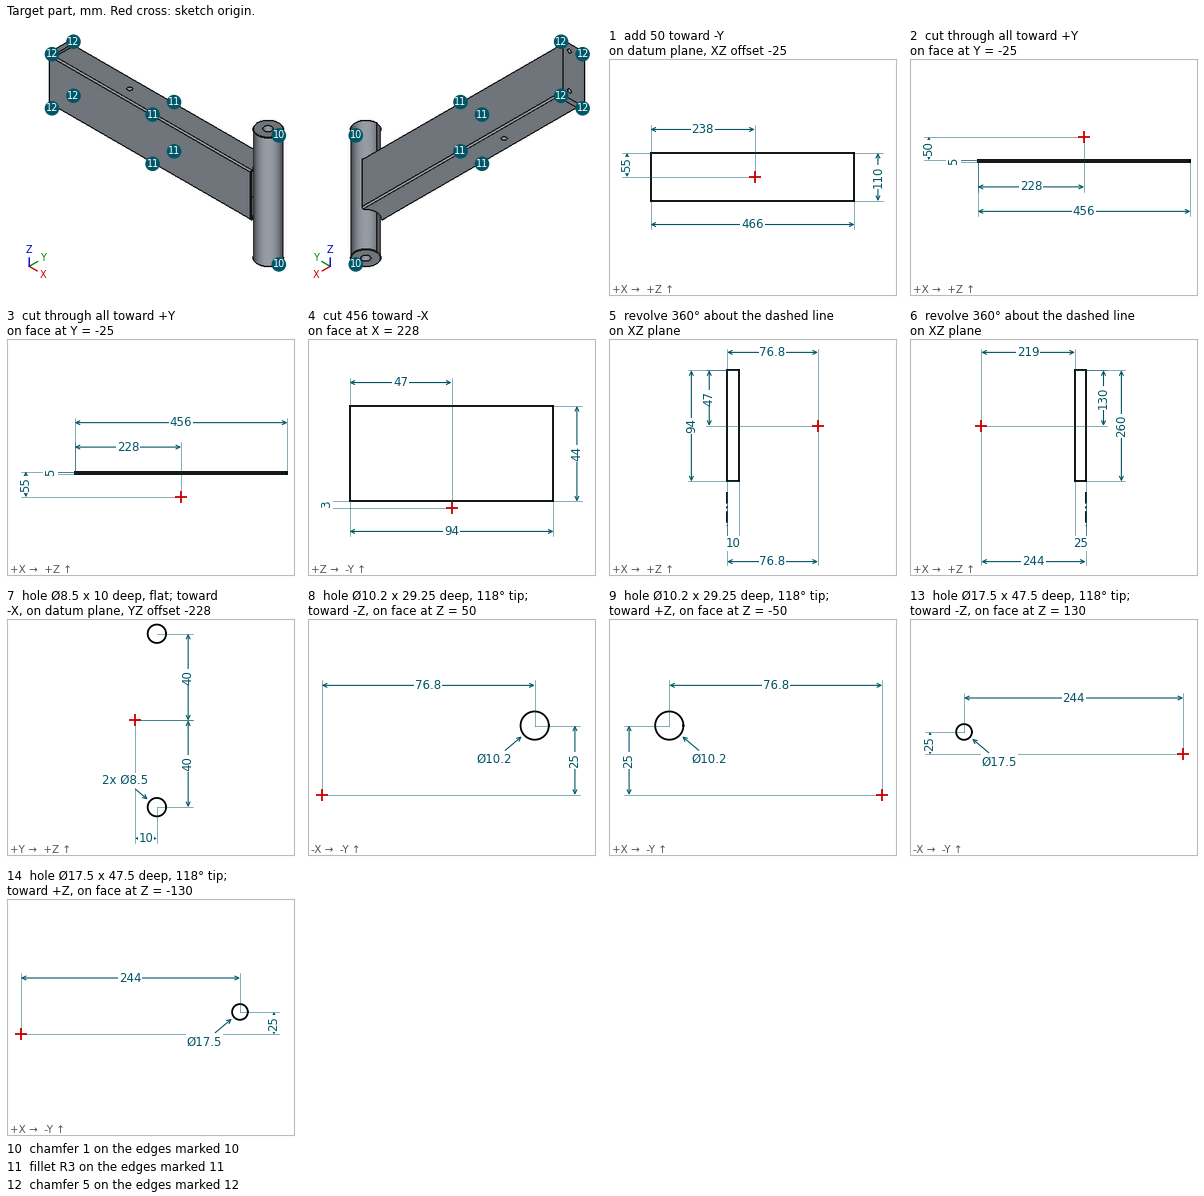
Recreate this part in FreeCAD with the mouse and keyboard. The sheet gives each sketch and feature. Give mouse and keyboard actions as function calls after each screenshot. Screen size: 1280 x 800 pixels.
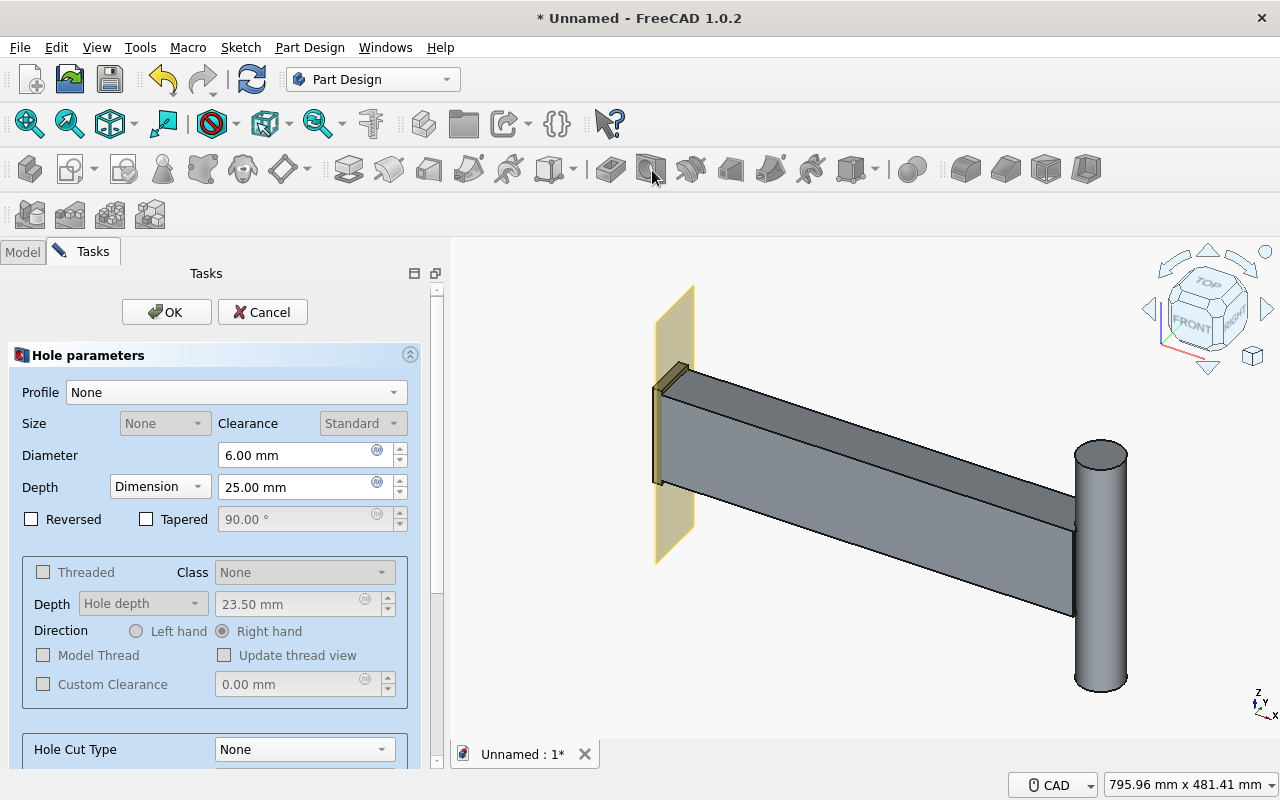
triple_click(305, 455)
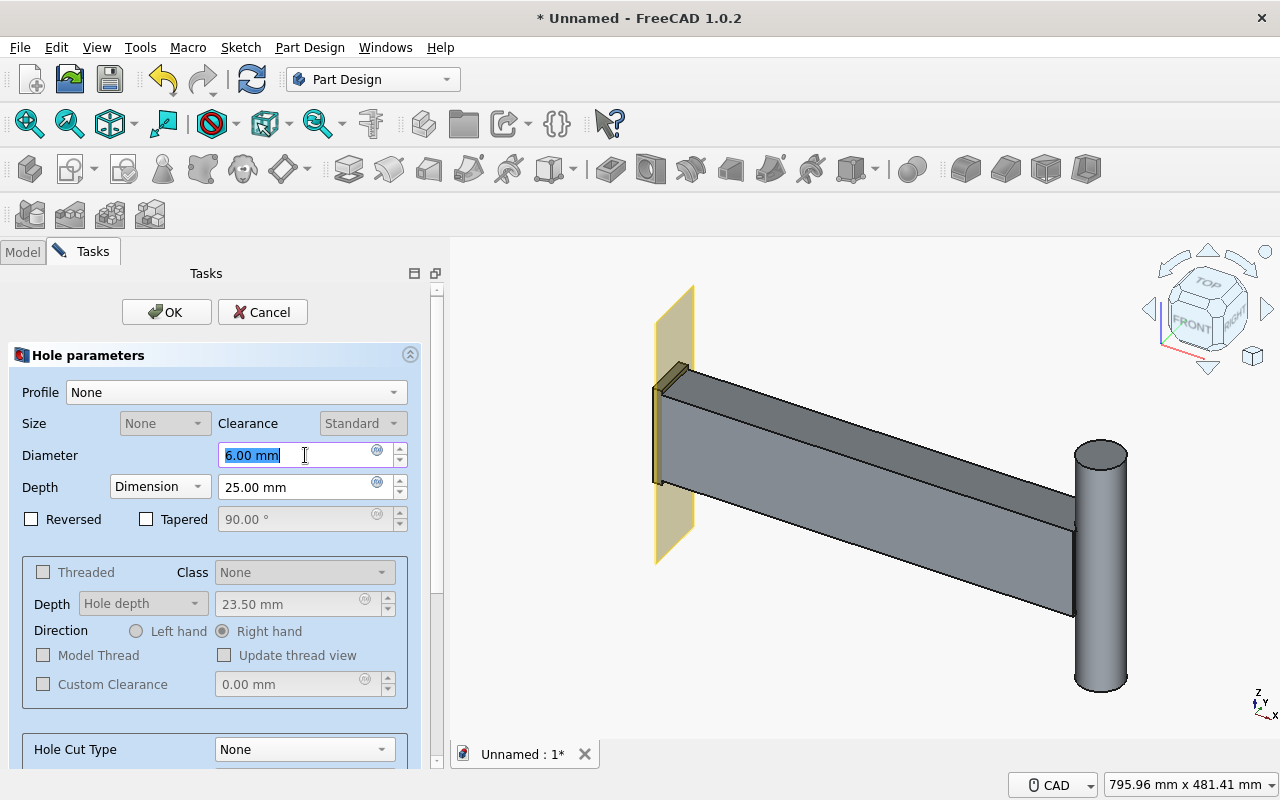
text(8.5)
key(Tab)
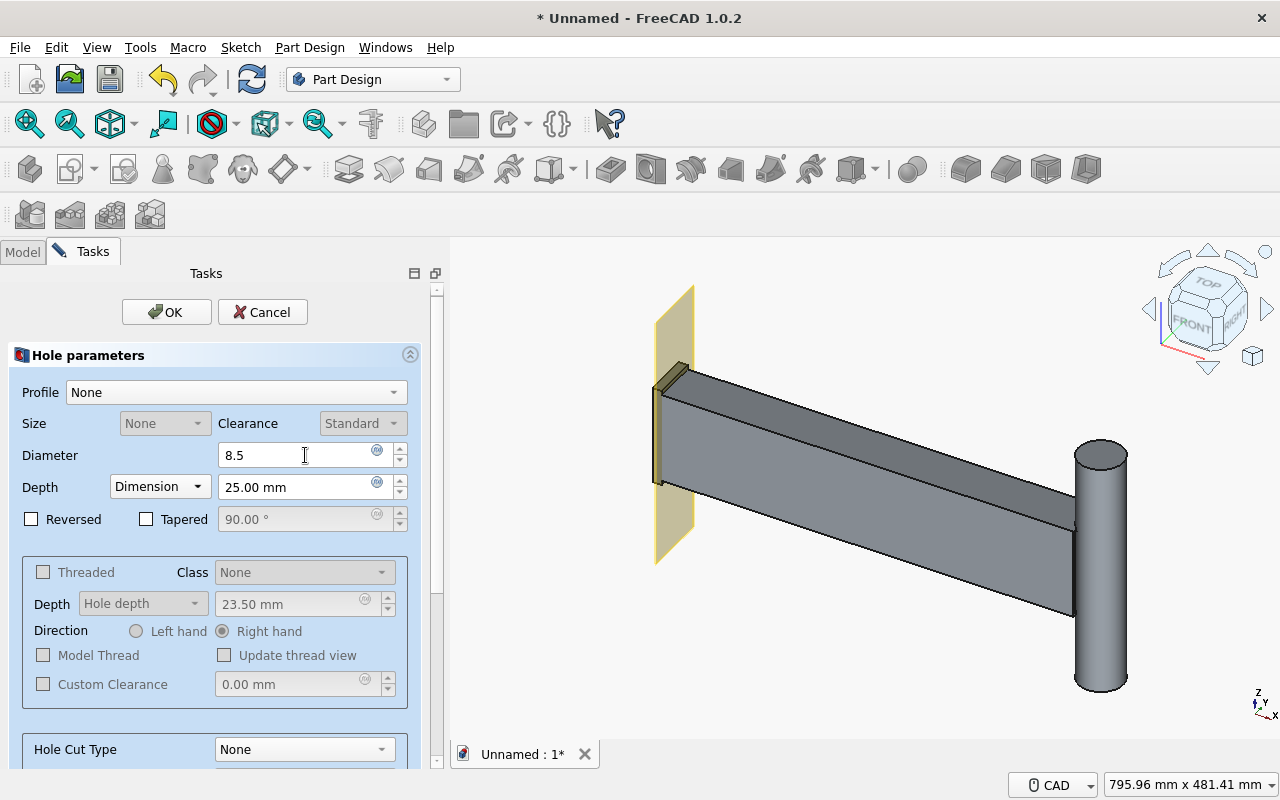
triple_click(305, 487)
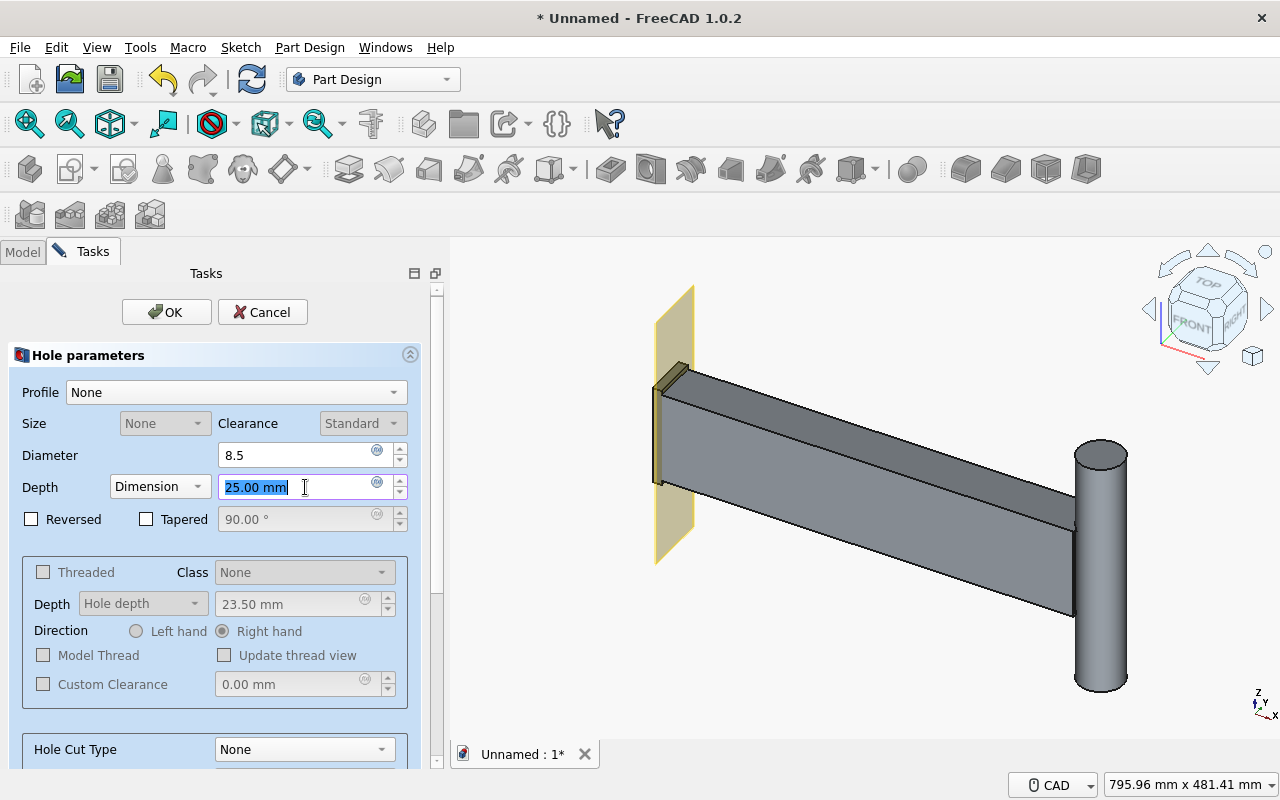
text(10)
key(Tab)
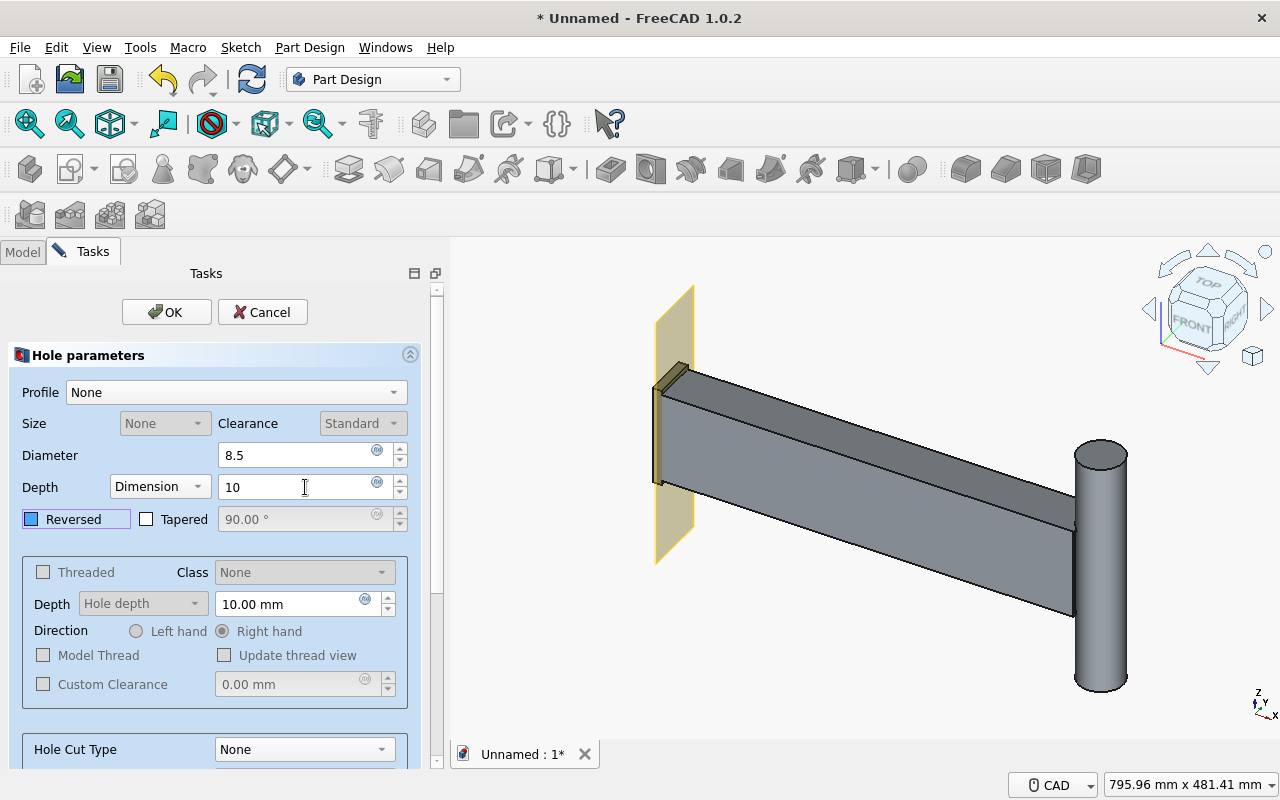
scroll(437, 526, down, 4)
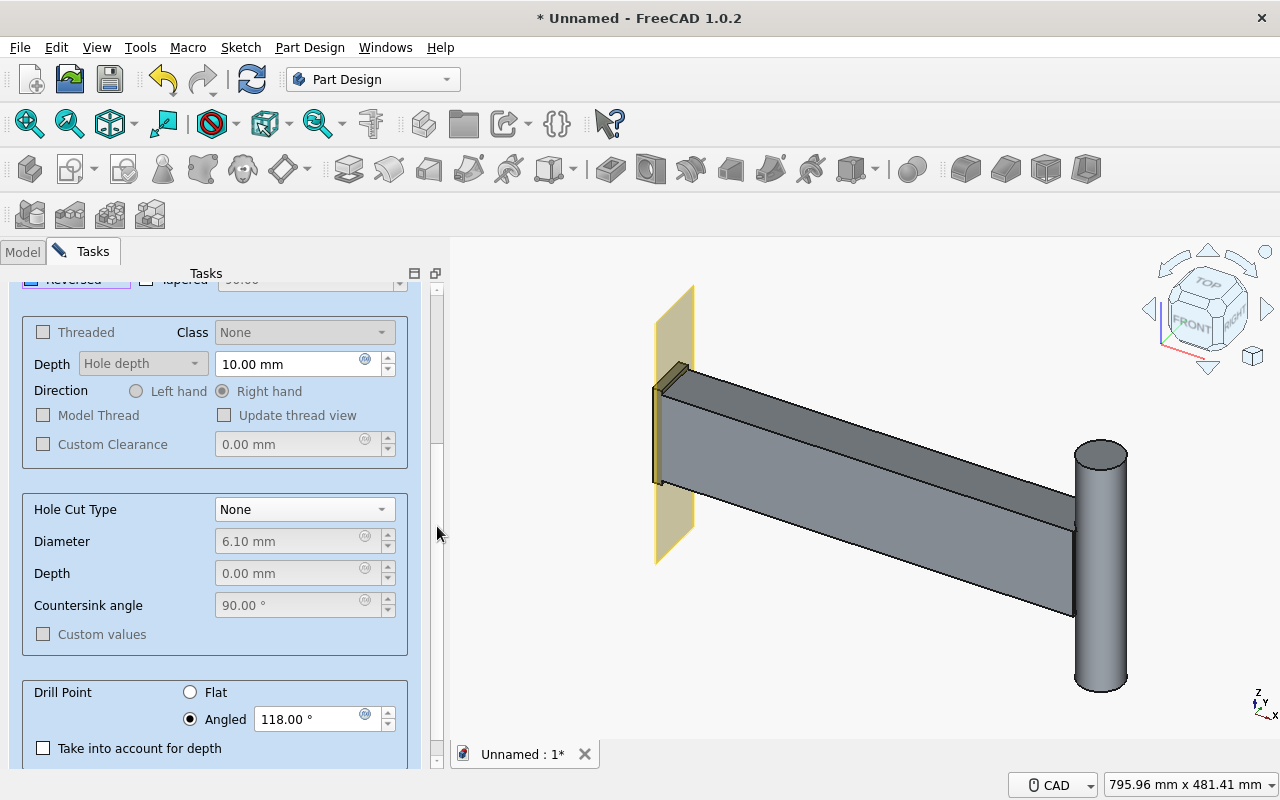
click(191, 692)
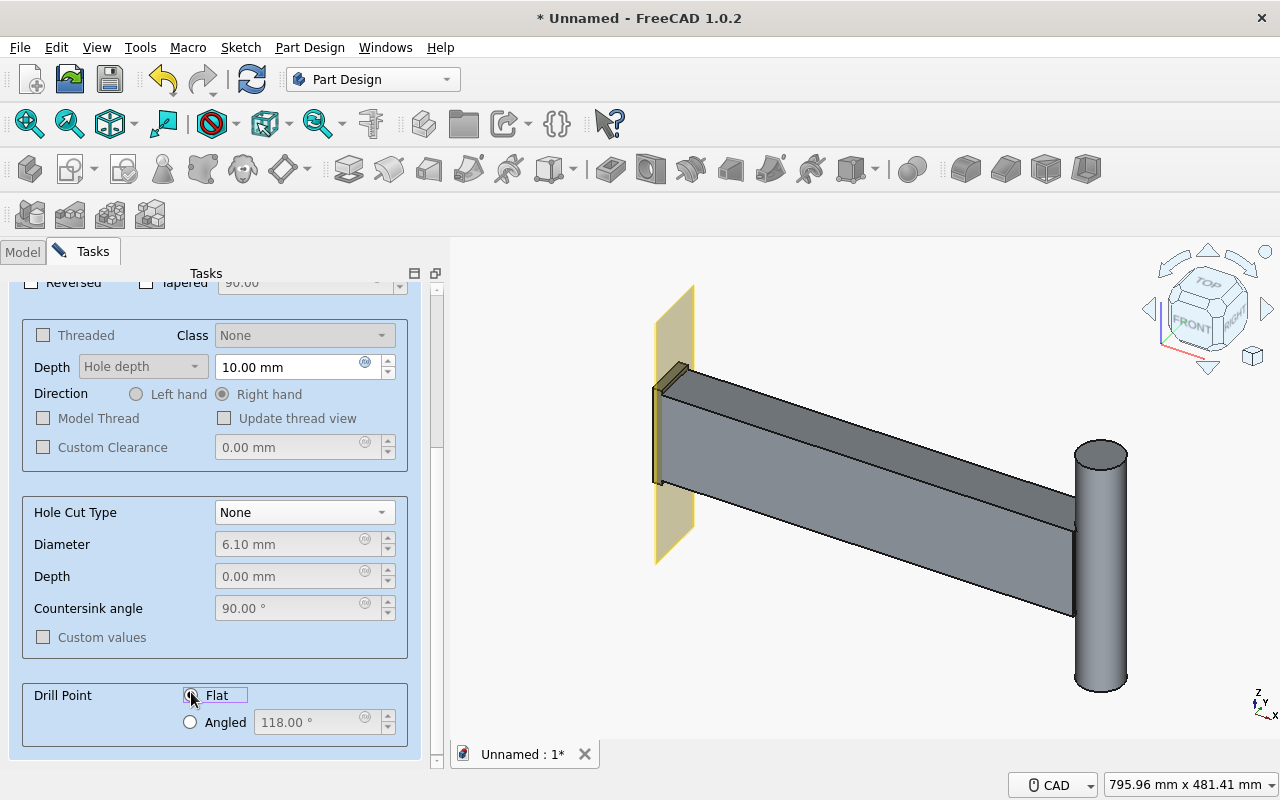
scroll(437, 526, up, 5)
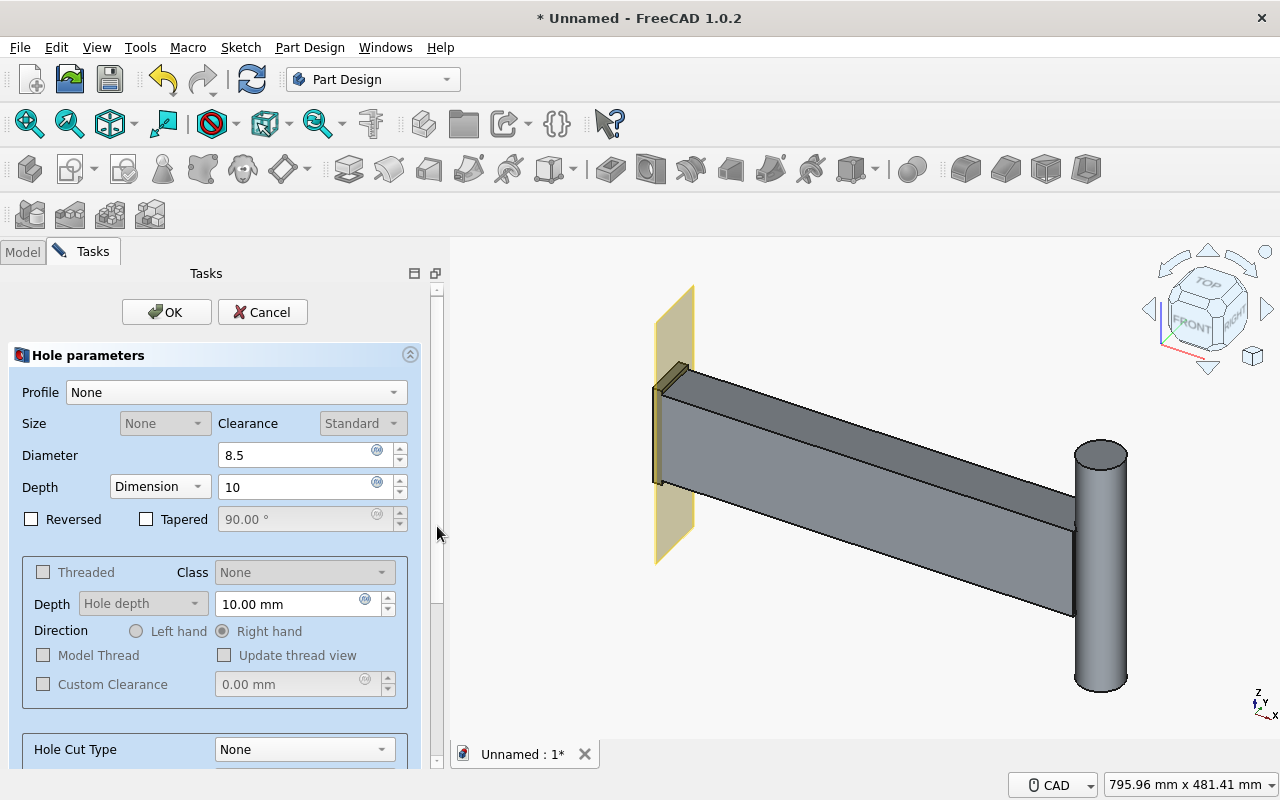
click(167, 312)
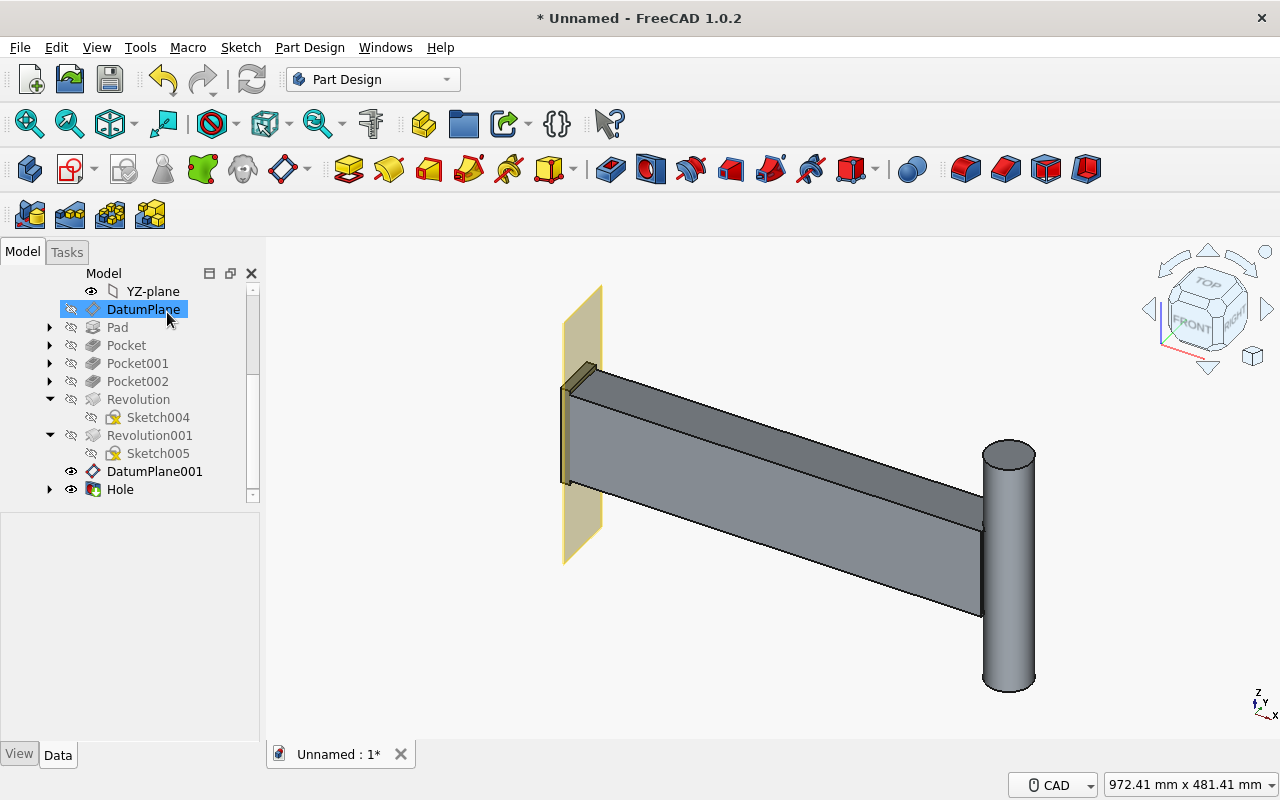
click(116, 471)
key(space)